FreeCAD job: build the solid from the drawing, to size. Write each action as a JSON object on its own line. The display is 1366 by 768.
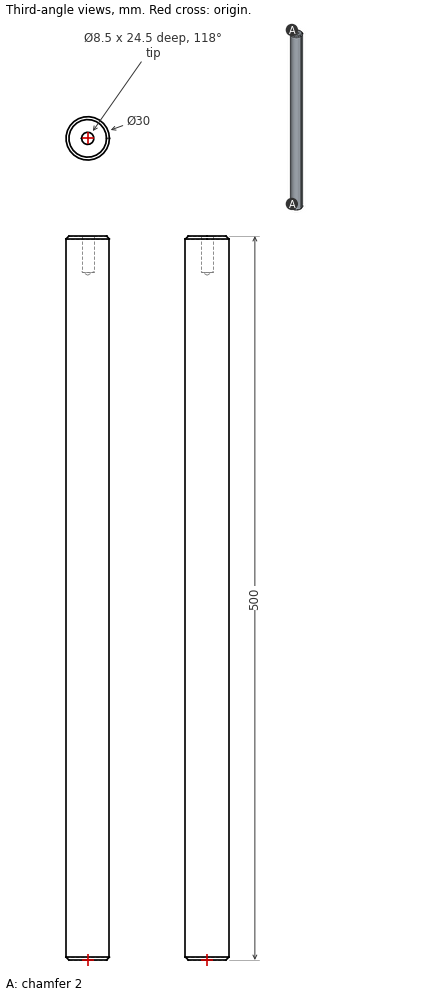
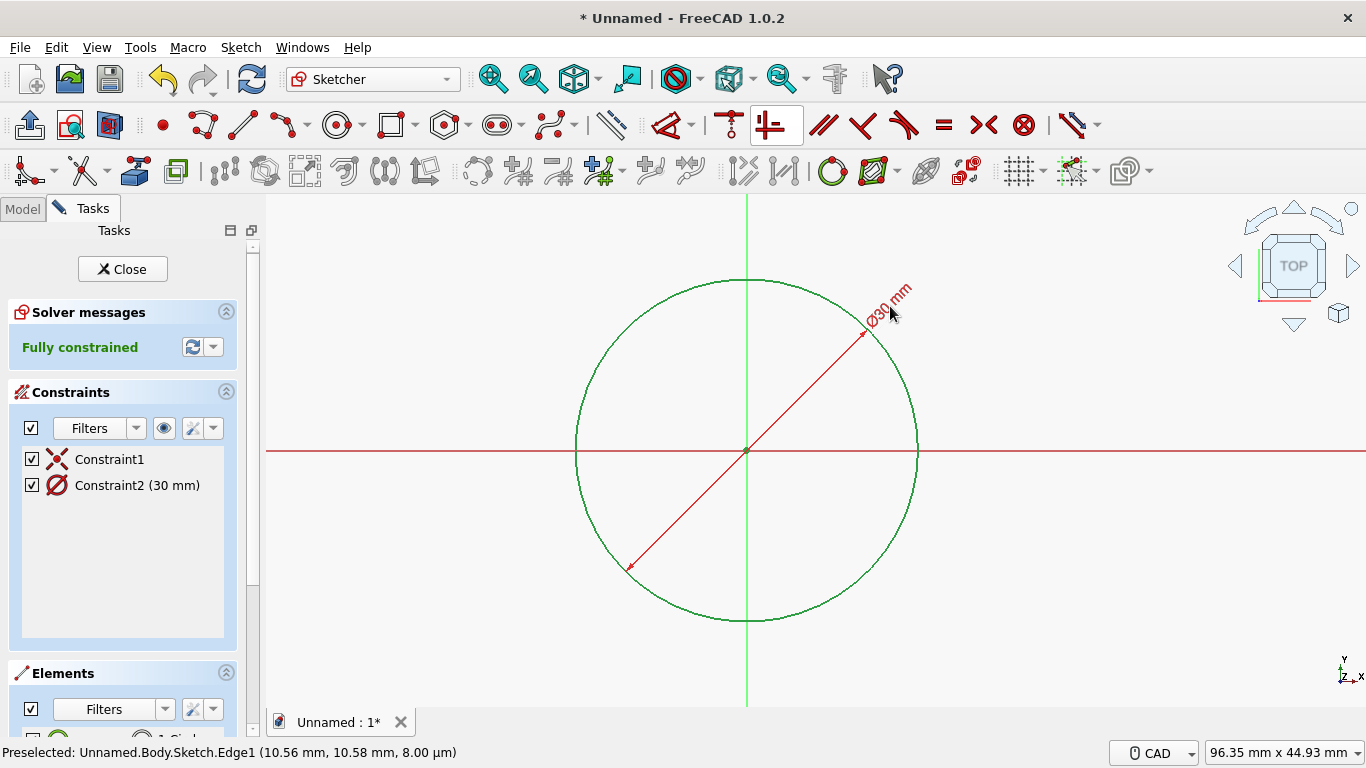
{"action": "left_click", "coordinate": [123, 269]}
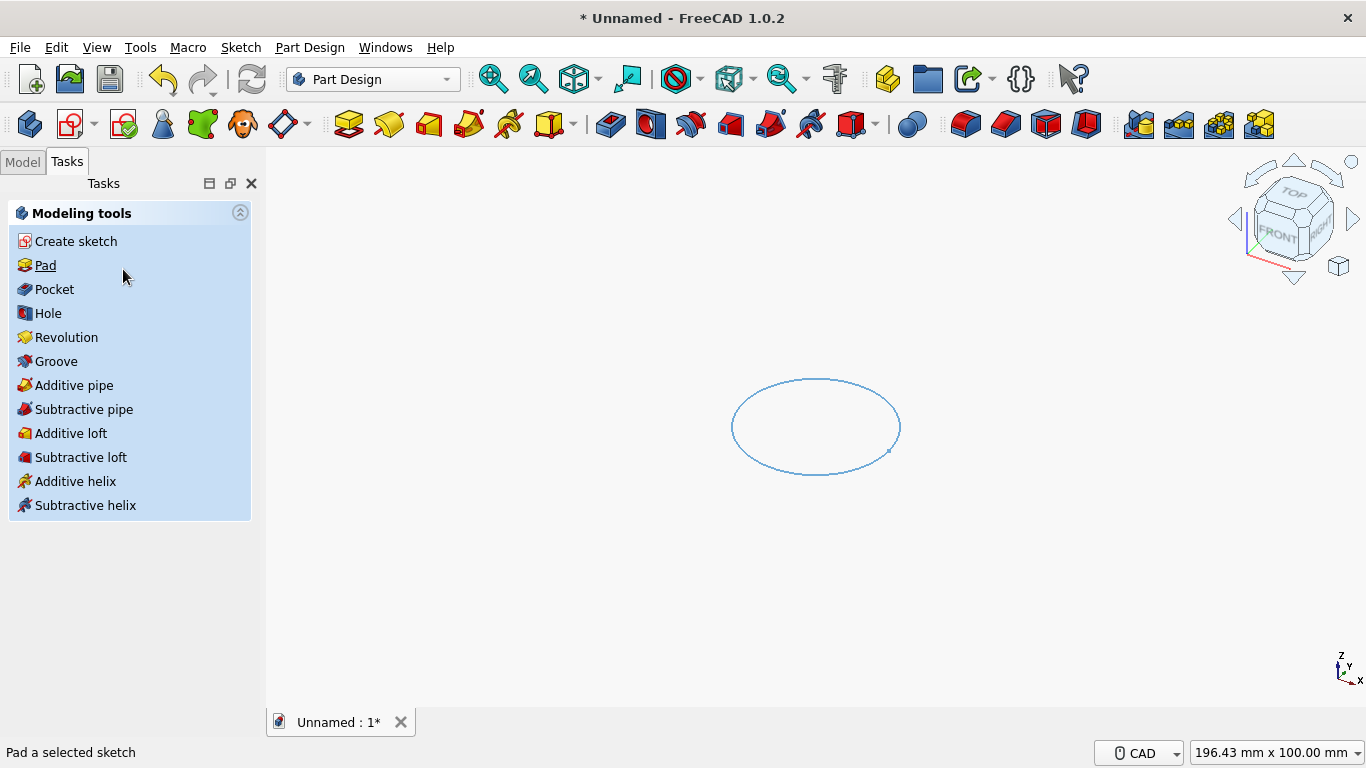
{"action": "left_click", "coordinate": [350, 124]}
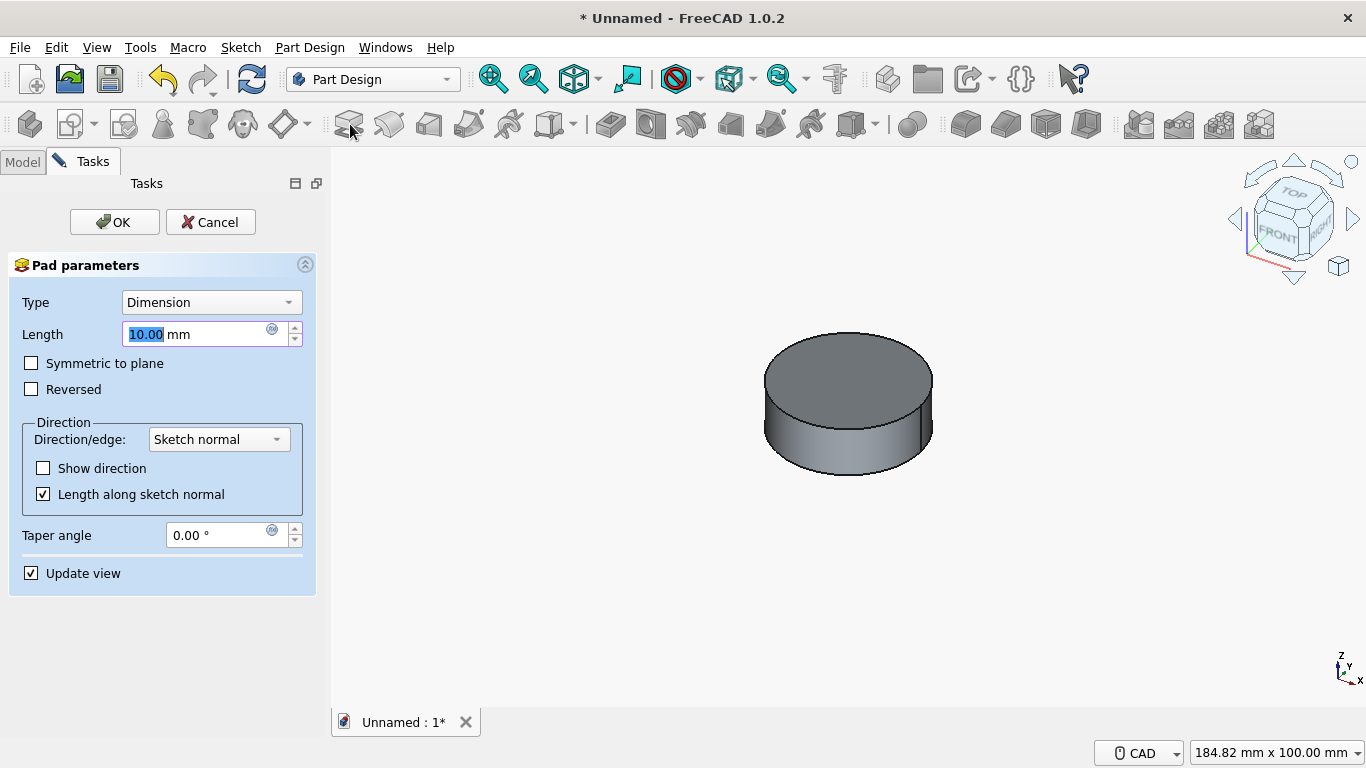
{"action": "type", "text": "500"}
{"action": "key", "text": "Tab"}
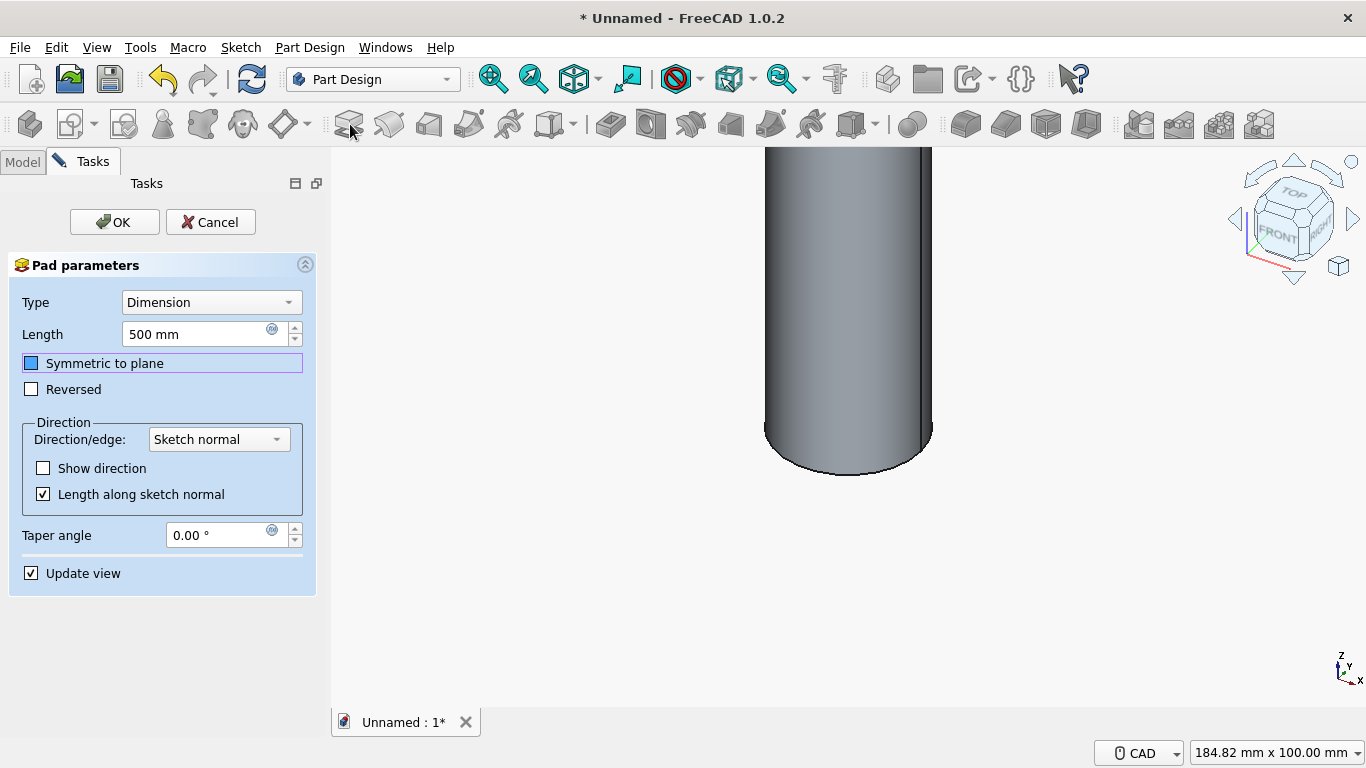
{"action": "left_click", "coordinate": [115, 222]}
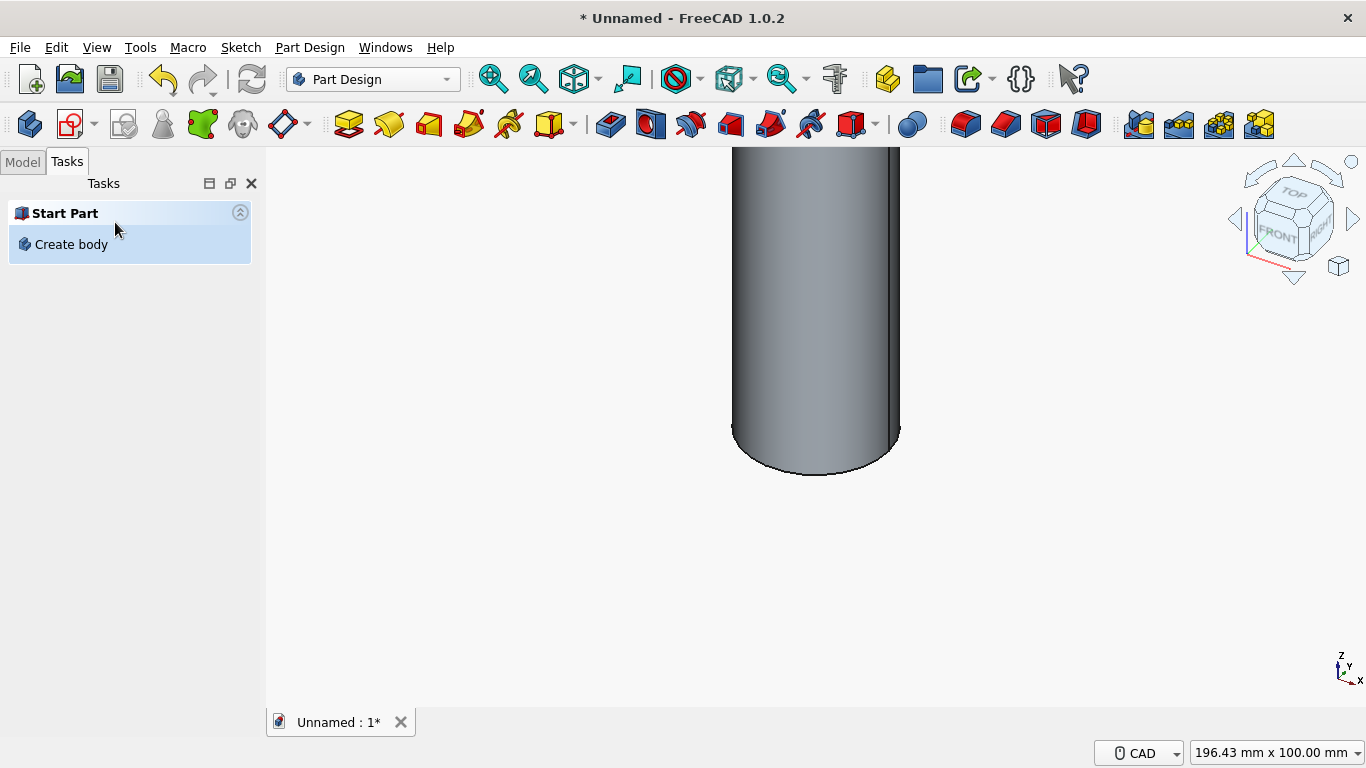
{"action": "left_click", "coordinate": [494, 80]}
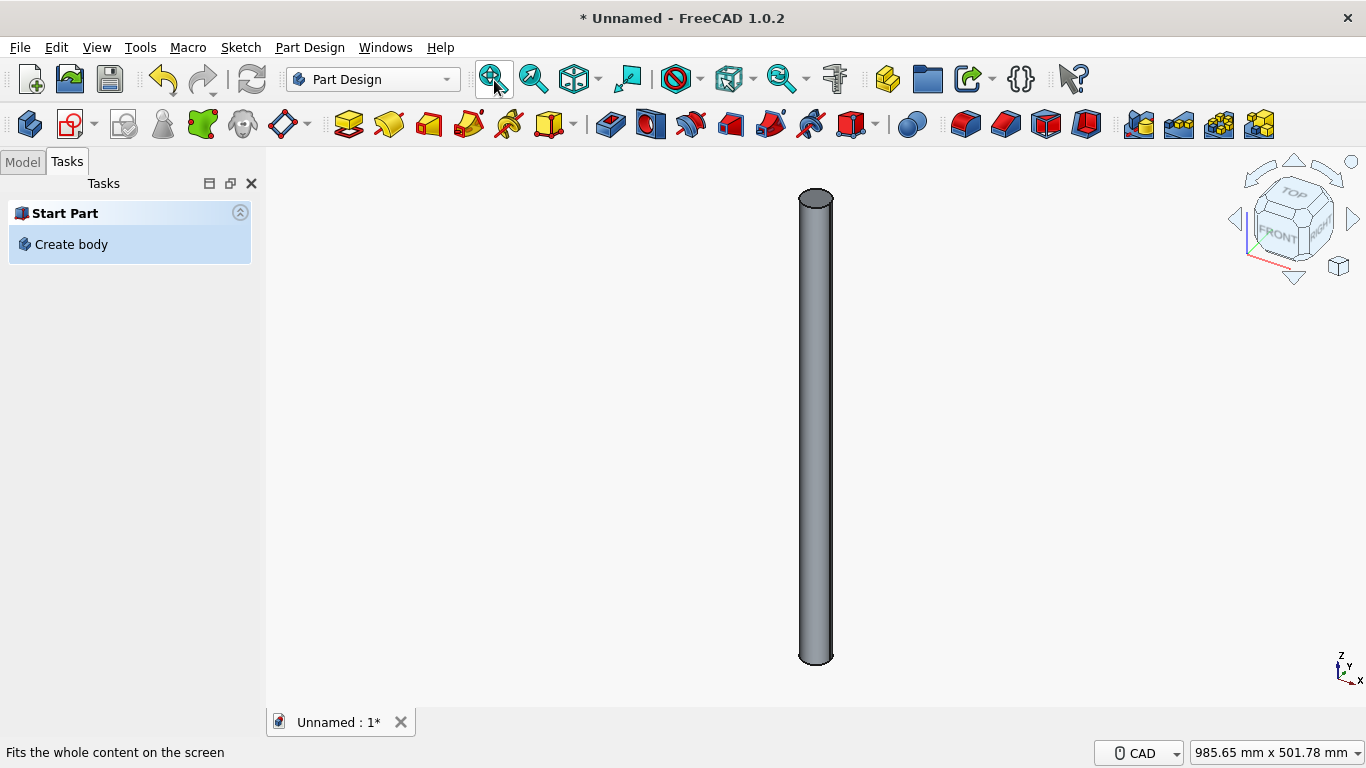
{"action": "left_click", "coordinate": [799, 656]}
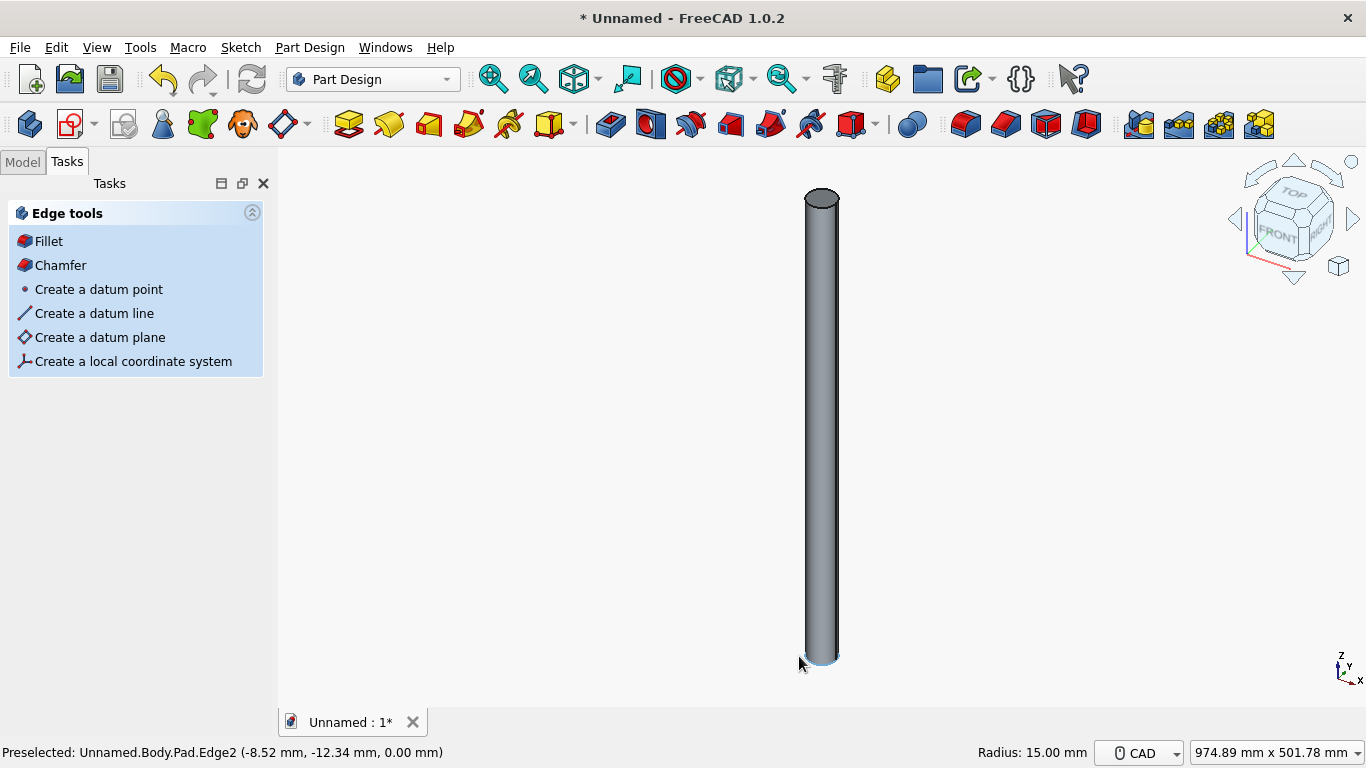
{"action": "left_click", "coordinate": [808, 193], "text": "ctrl"}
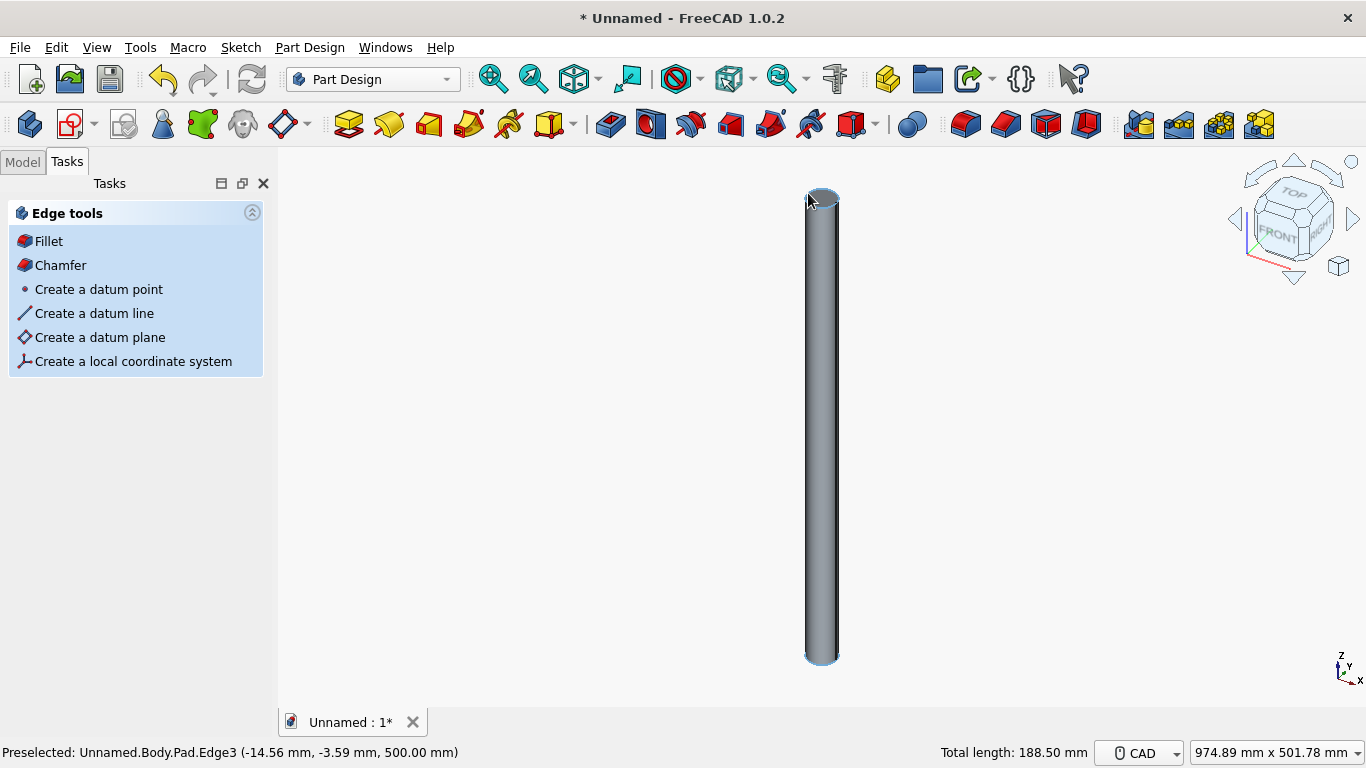
{"action": "left_click", "coordinate": [1006, 124]}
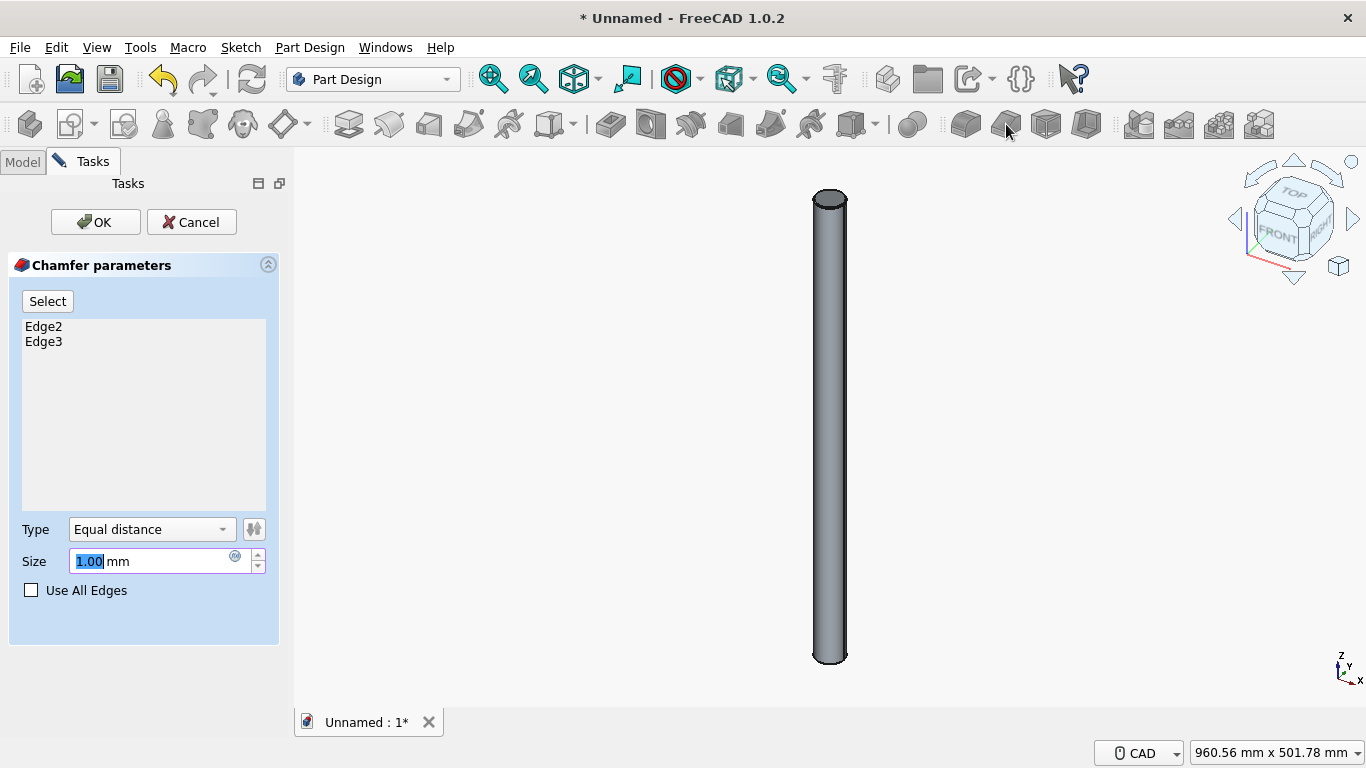
{"action": "type", "text": "2"}
{"action": "key", "text": "Tab"}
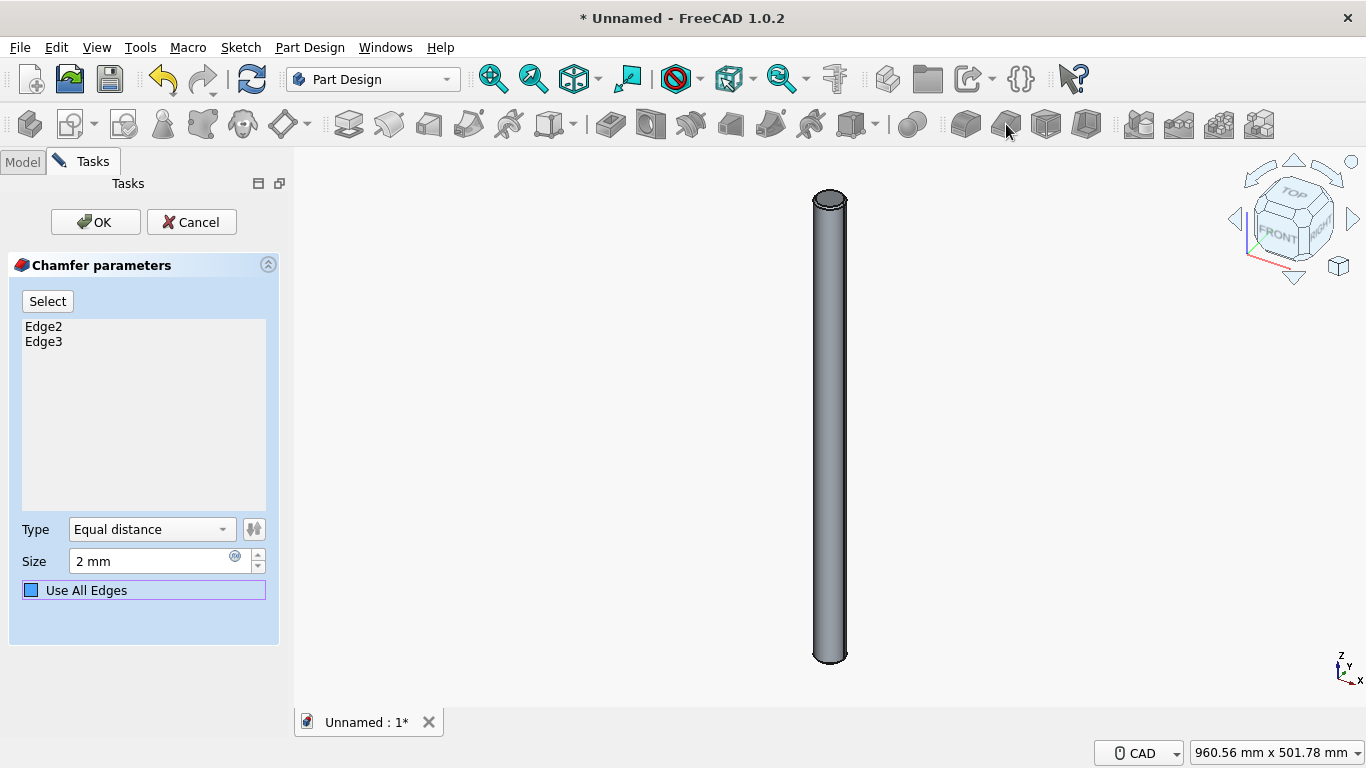
{"action": "left_click", "coordinate": [96, 222]}